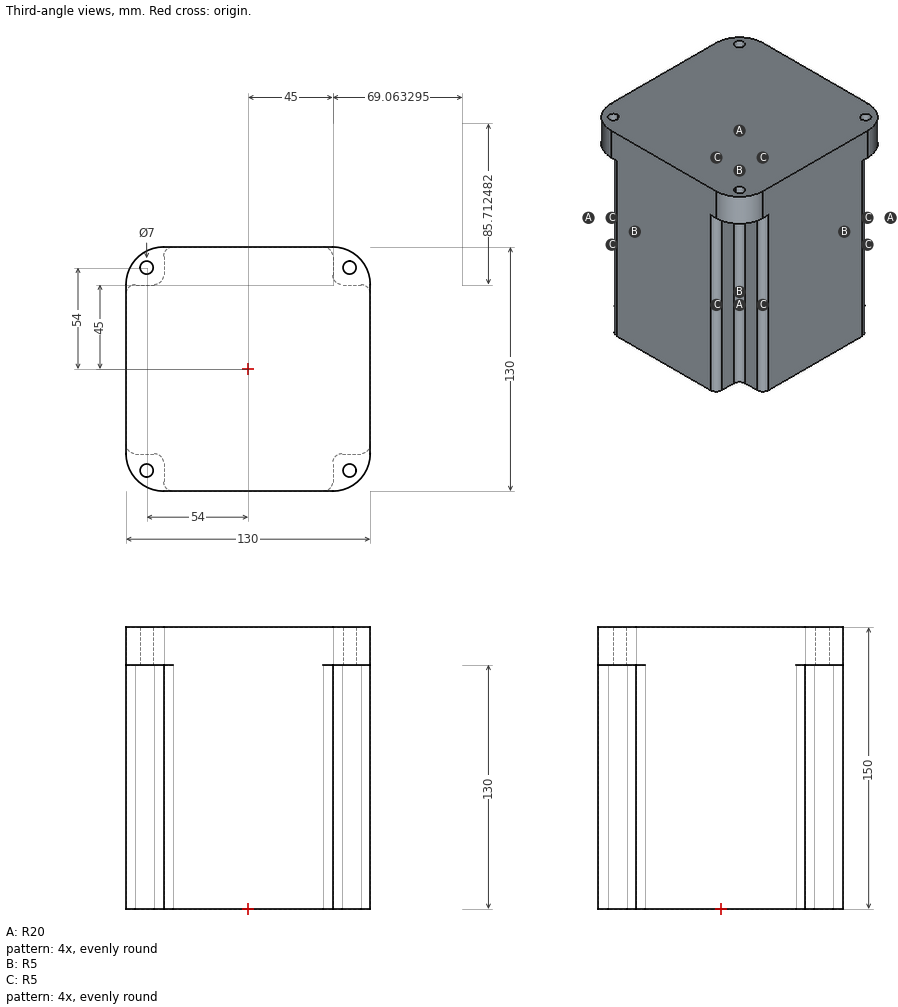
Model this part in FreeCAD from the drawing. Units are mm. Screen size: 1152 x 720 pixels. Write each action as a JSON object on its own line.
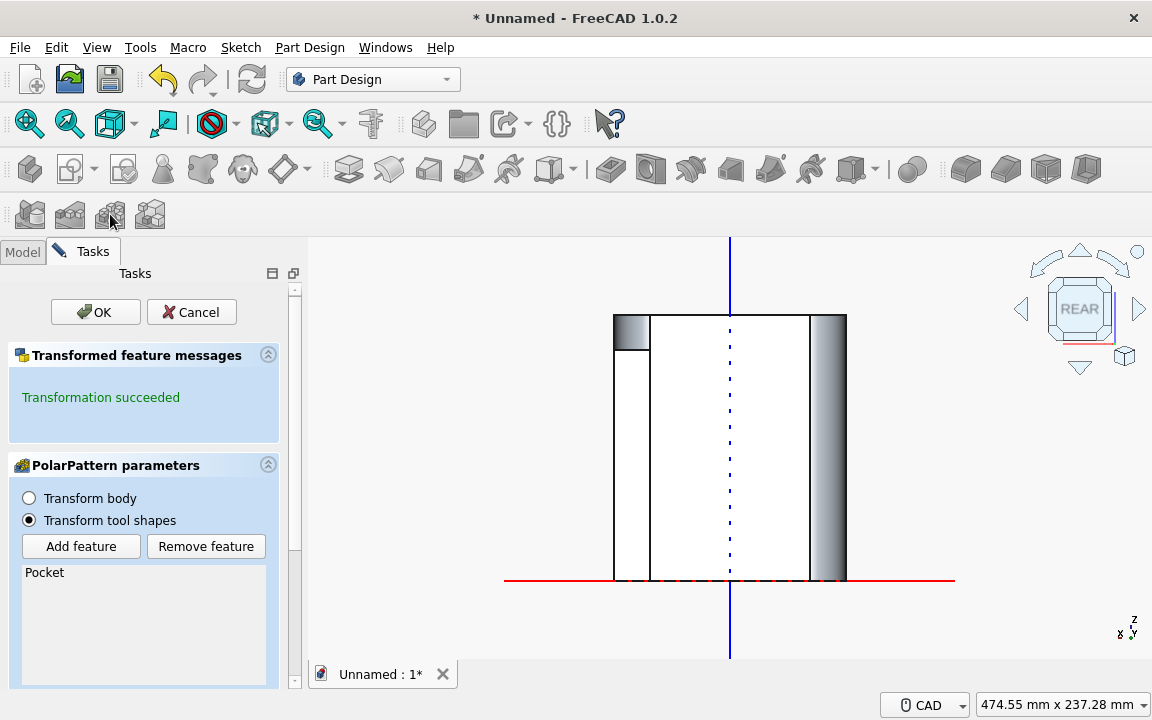
{"action": "scroll", "coordinate": [295, 486], "scroll_direction": "down", "scroll_amount": 2}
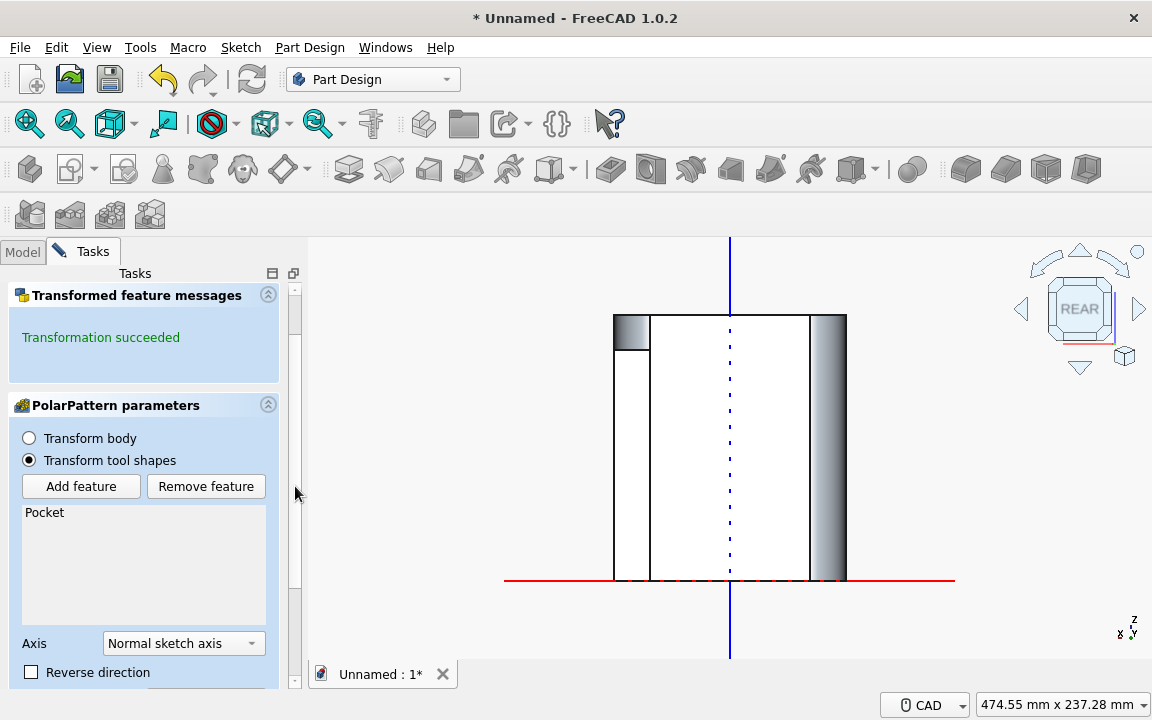
{"action": "left_click", "coordinate": [184, 584]}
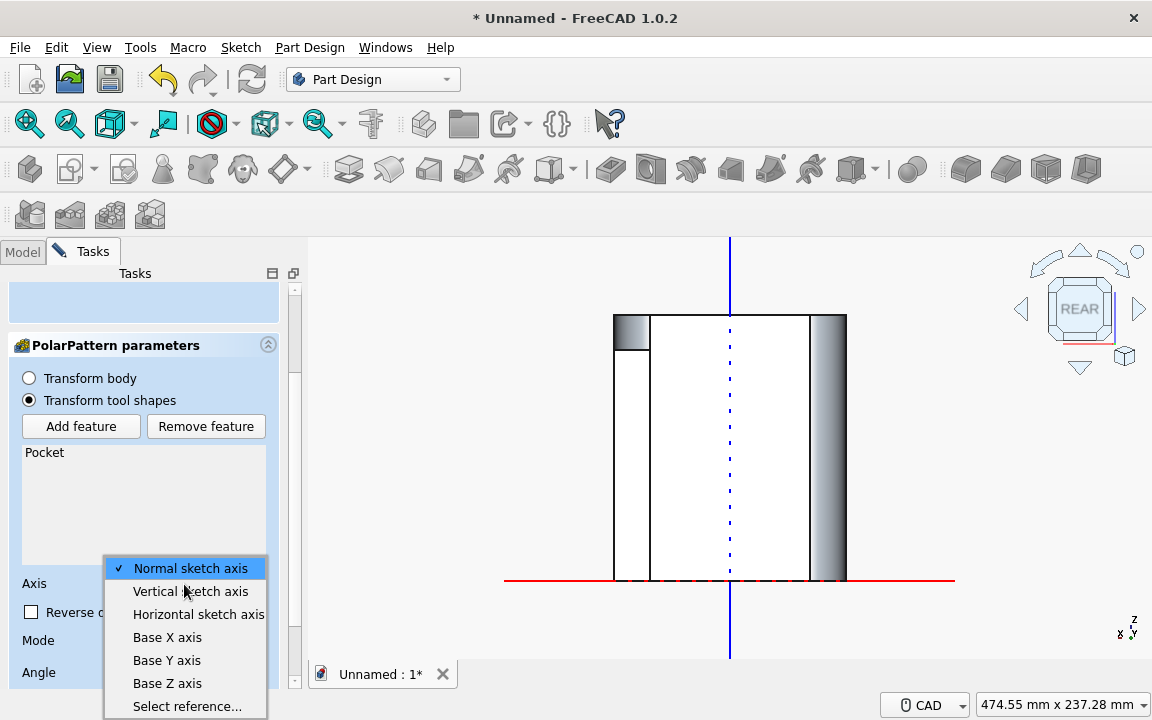
{"action": "left_click", "coordinate": [184, 684]}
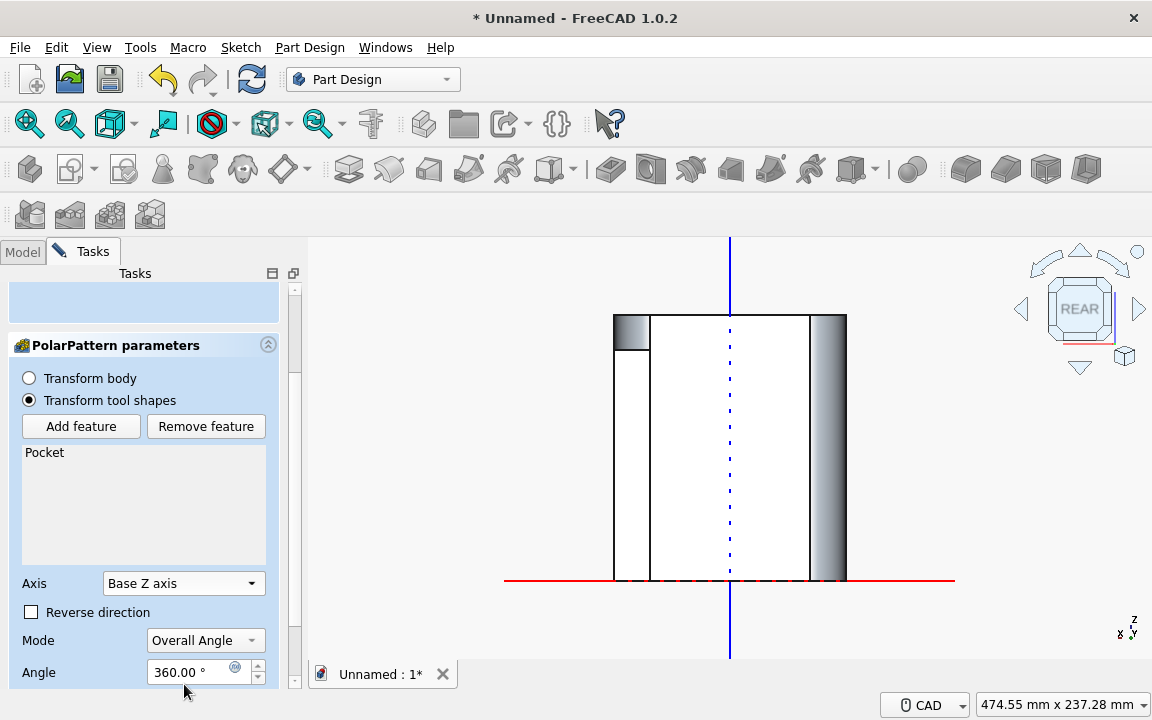
{"action": "scroll", "coordinate": [295, 486], "scroll_direction": "down", "scroll_amount": 2}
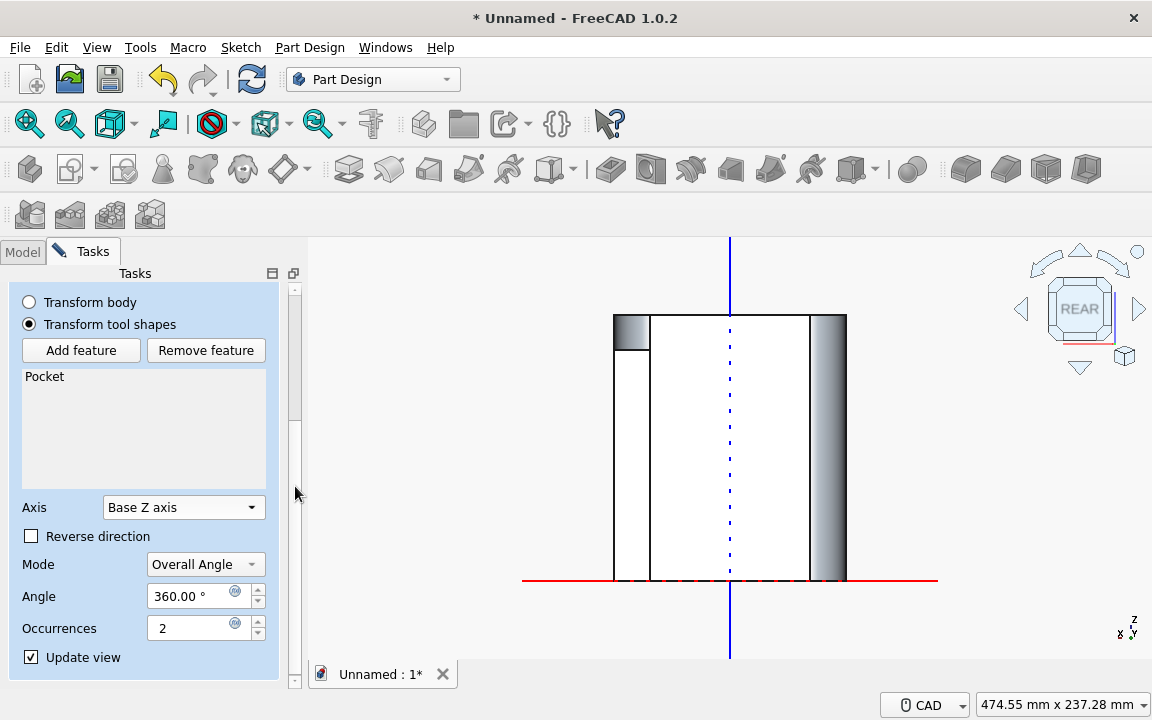
{"action": "triple_click", "coordinate": [198, 628]}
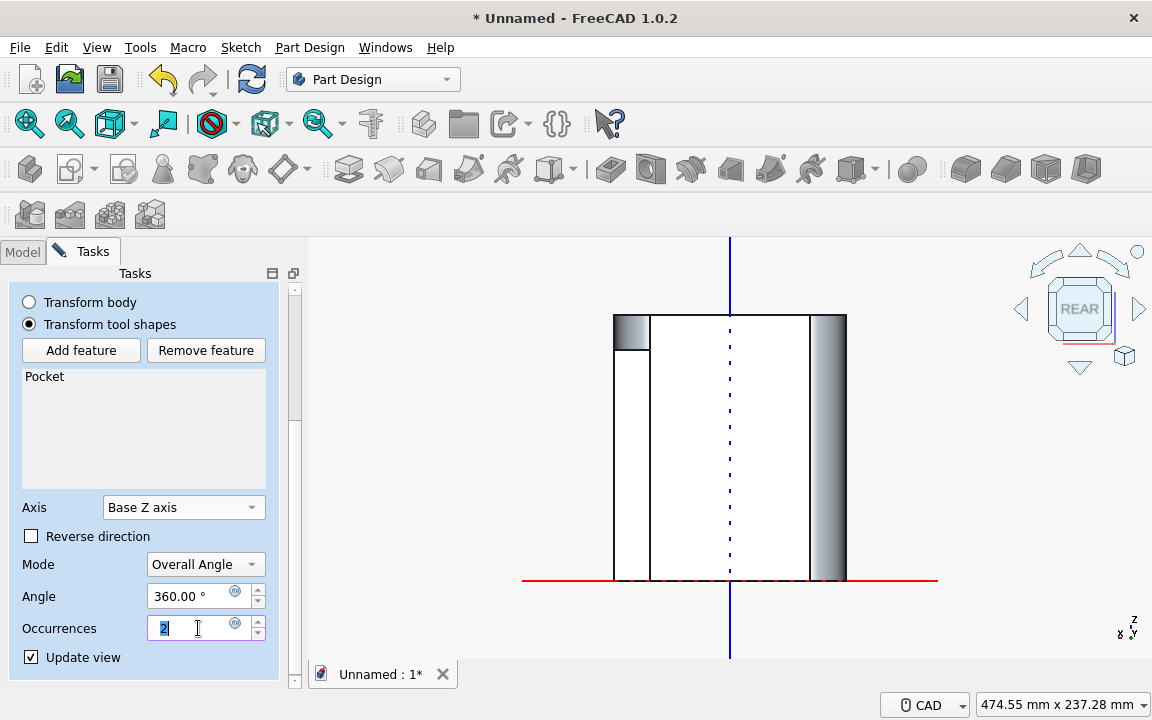
{"action": "type", "text": "4"}
{"action": "key", "text": "Tab"}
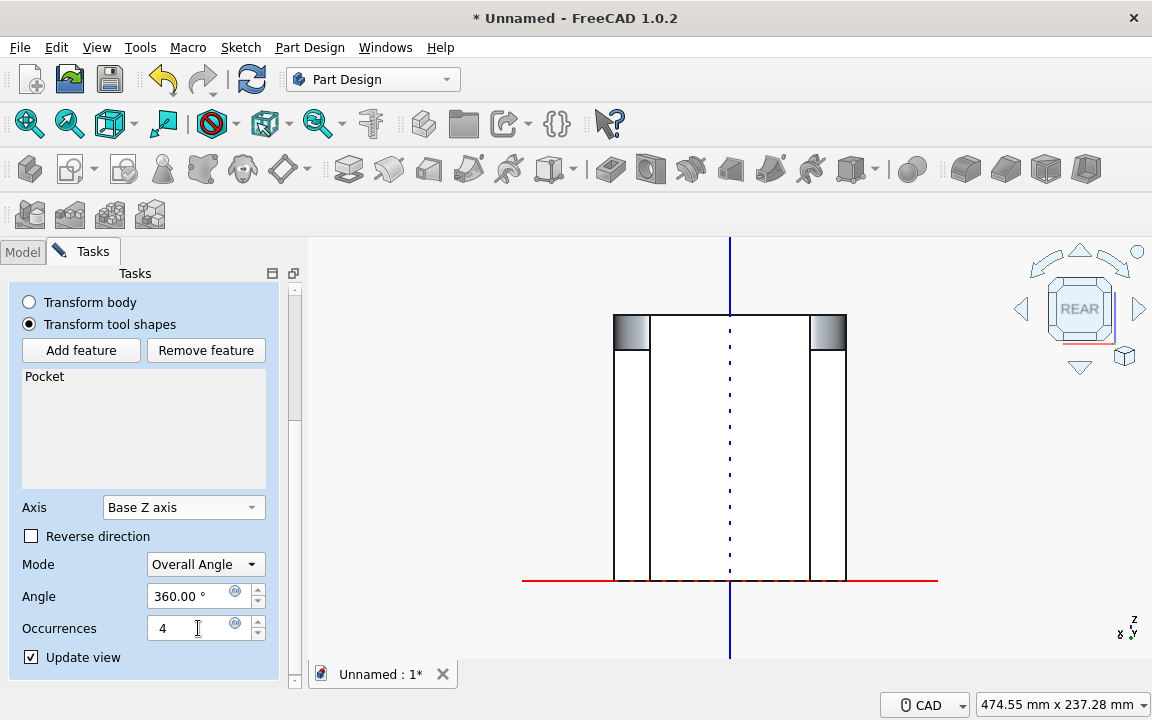
{"action": "scroll", "coordinate": [295, 486], "scroll_direction": "up", "scroll_amount": 5}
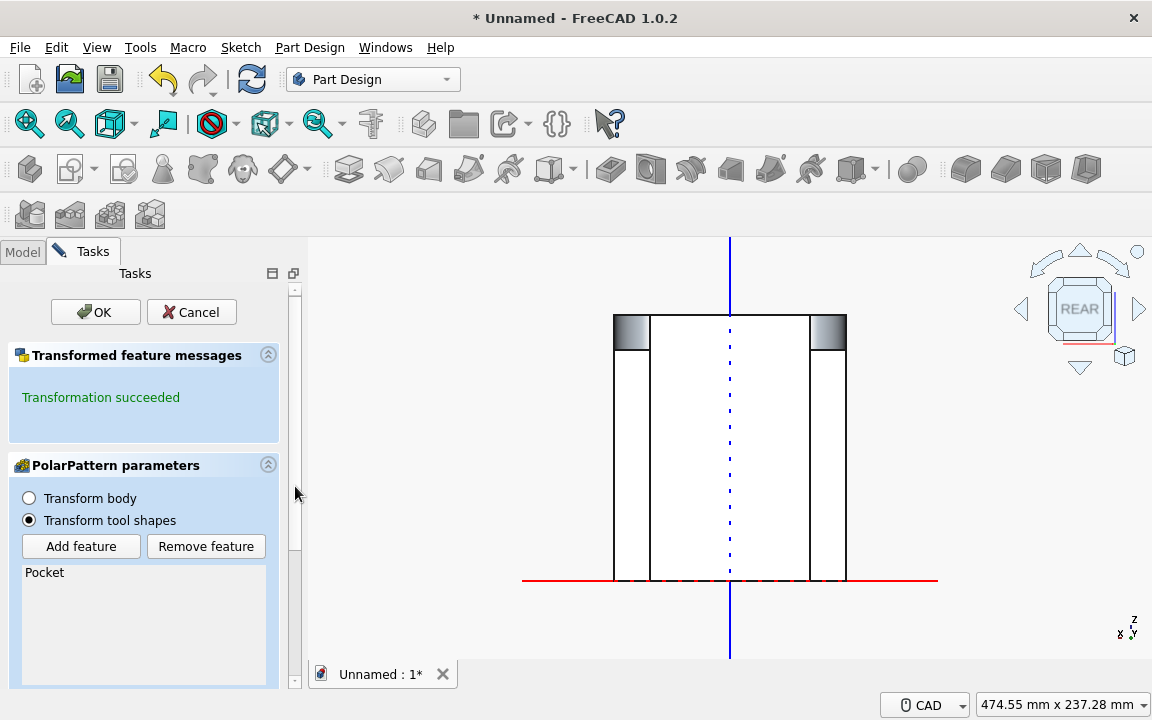
{"action": "left_click", "coordinate": [96, 312]}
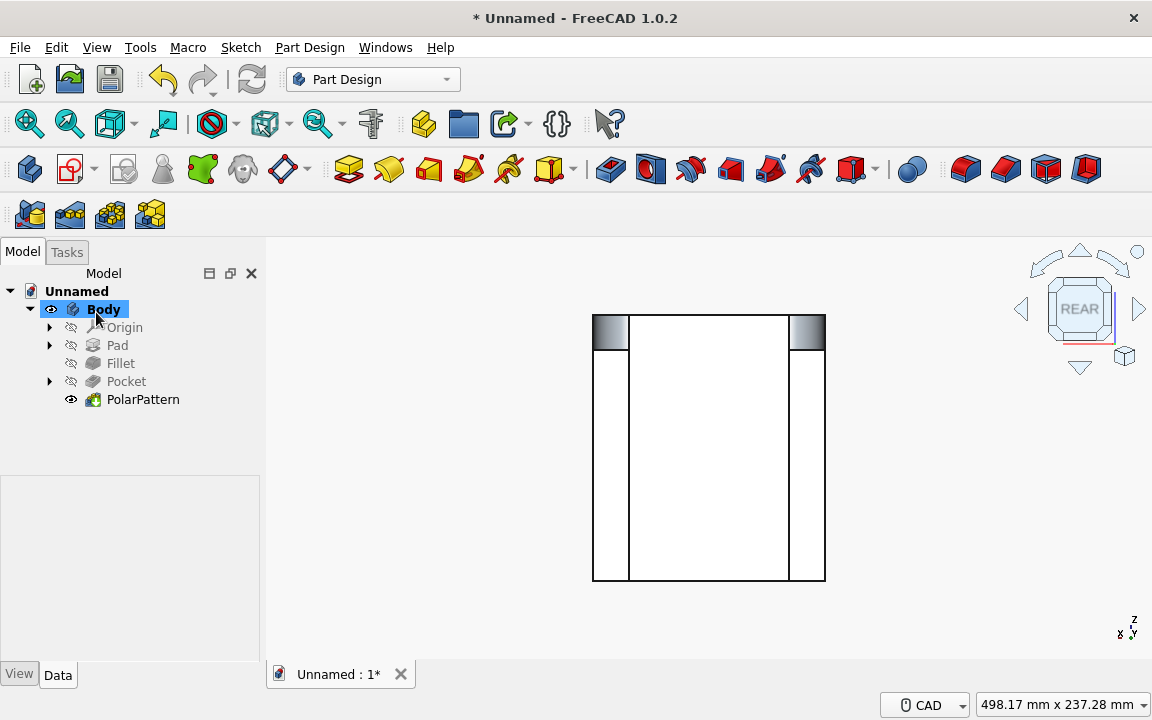
{"action": "key", "text": "0"}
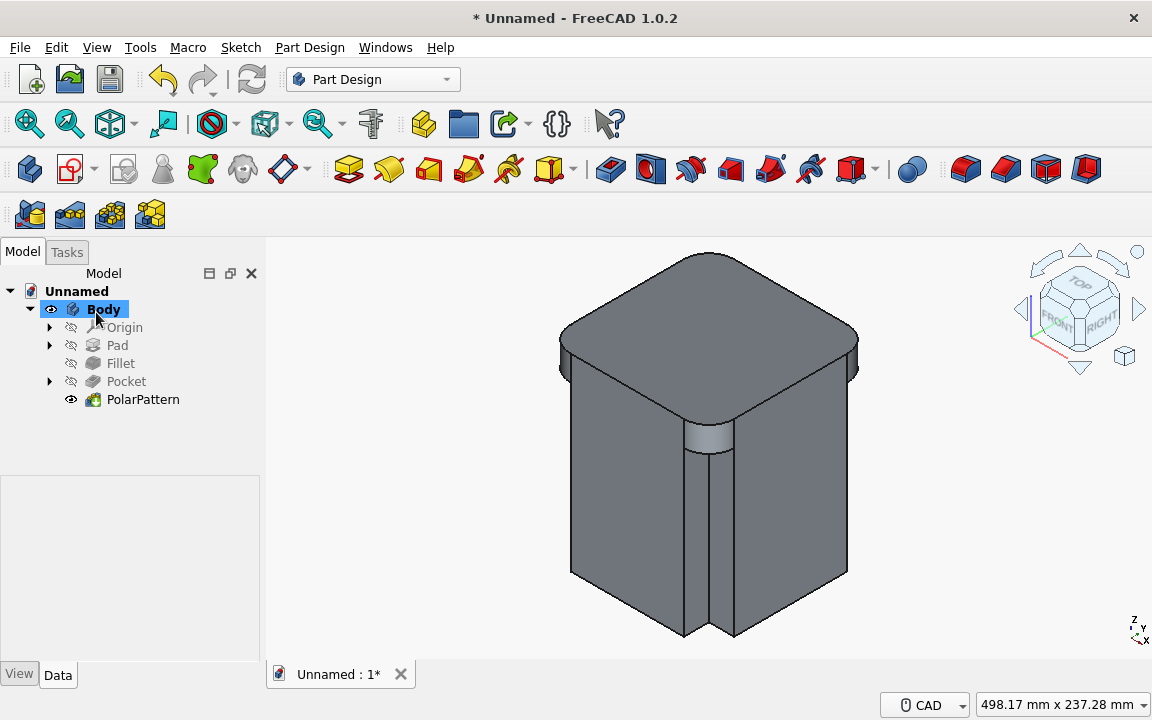
{"action": "key", "text": "2"}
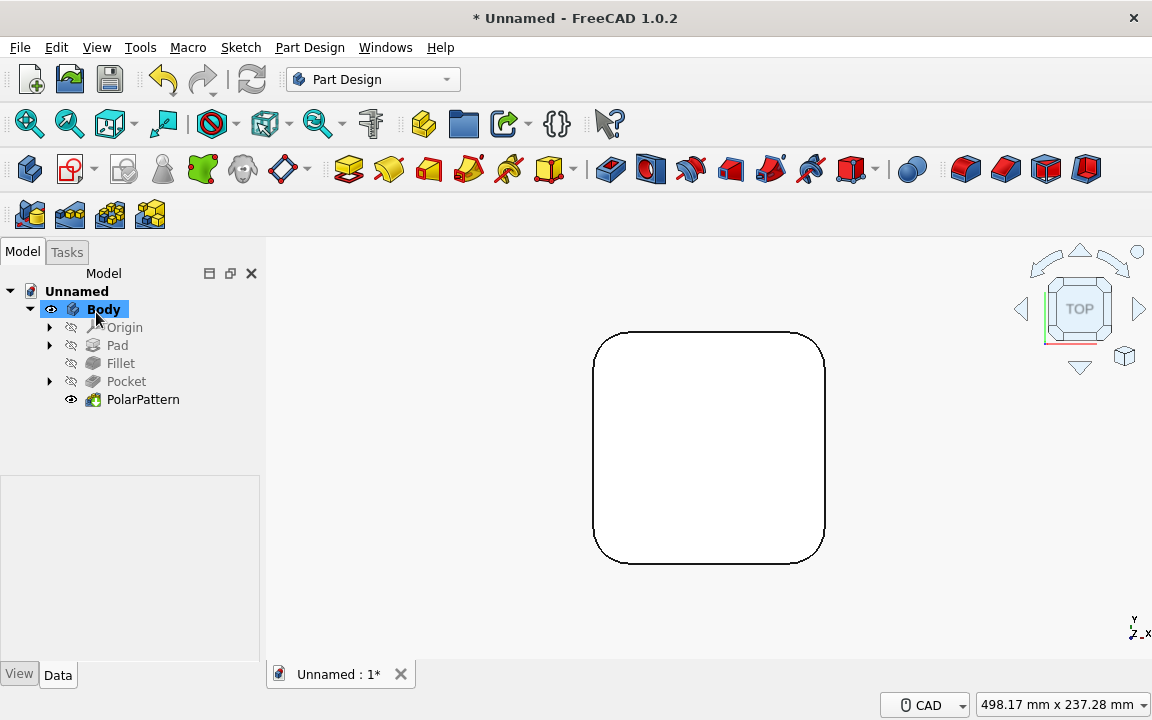
{"action": "key", "text": "1"}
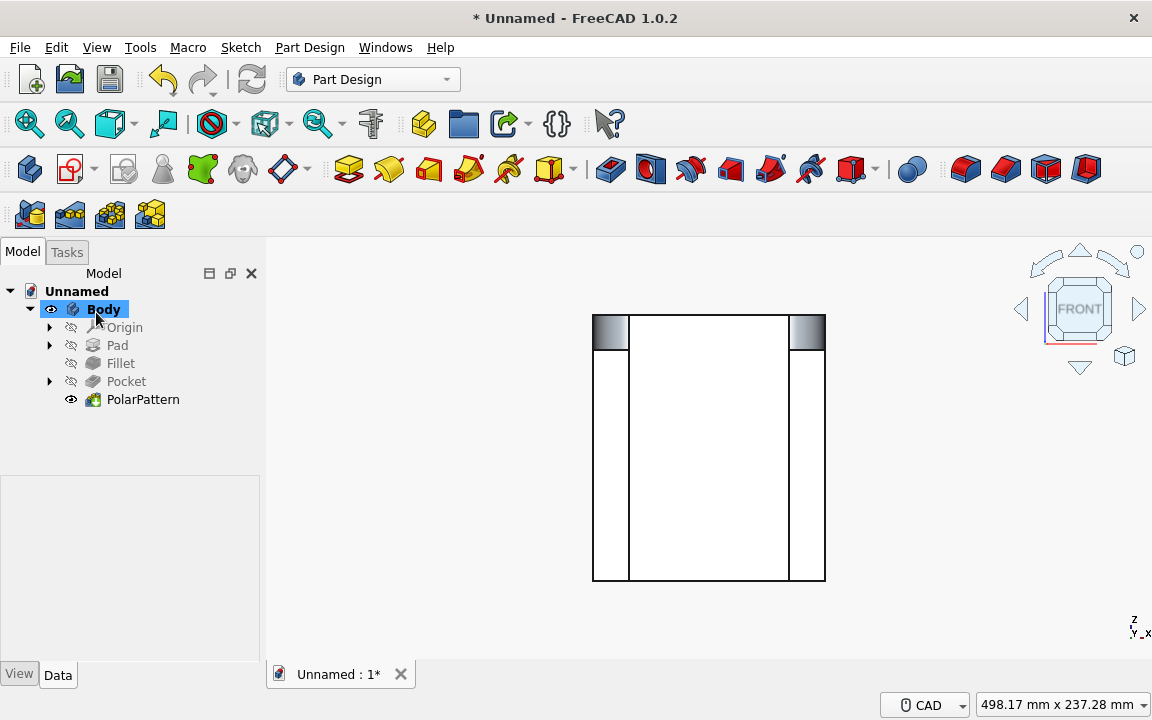
{"action": "key", "text": "3"}